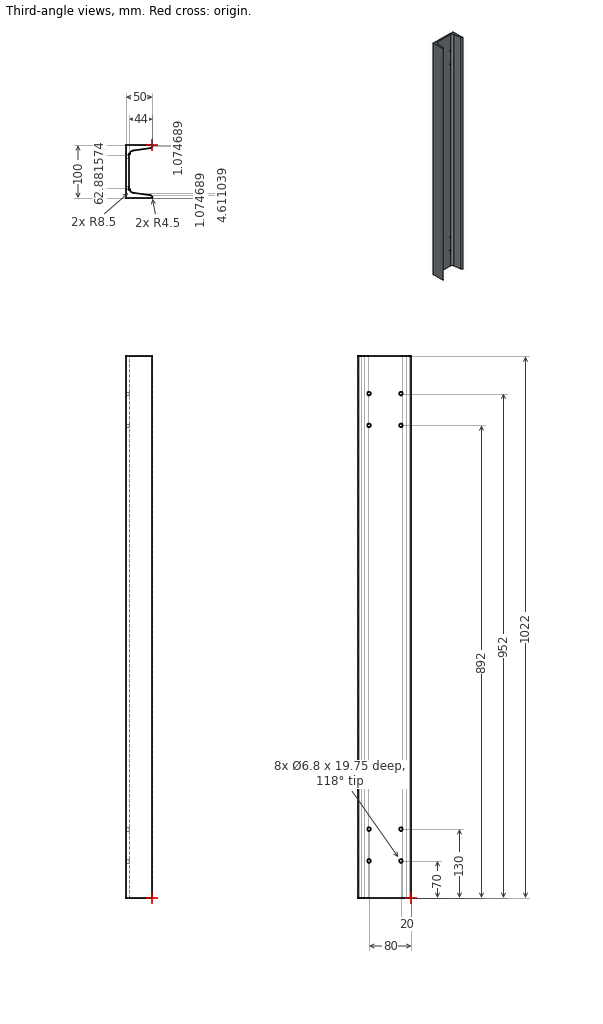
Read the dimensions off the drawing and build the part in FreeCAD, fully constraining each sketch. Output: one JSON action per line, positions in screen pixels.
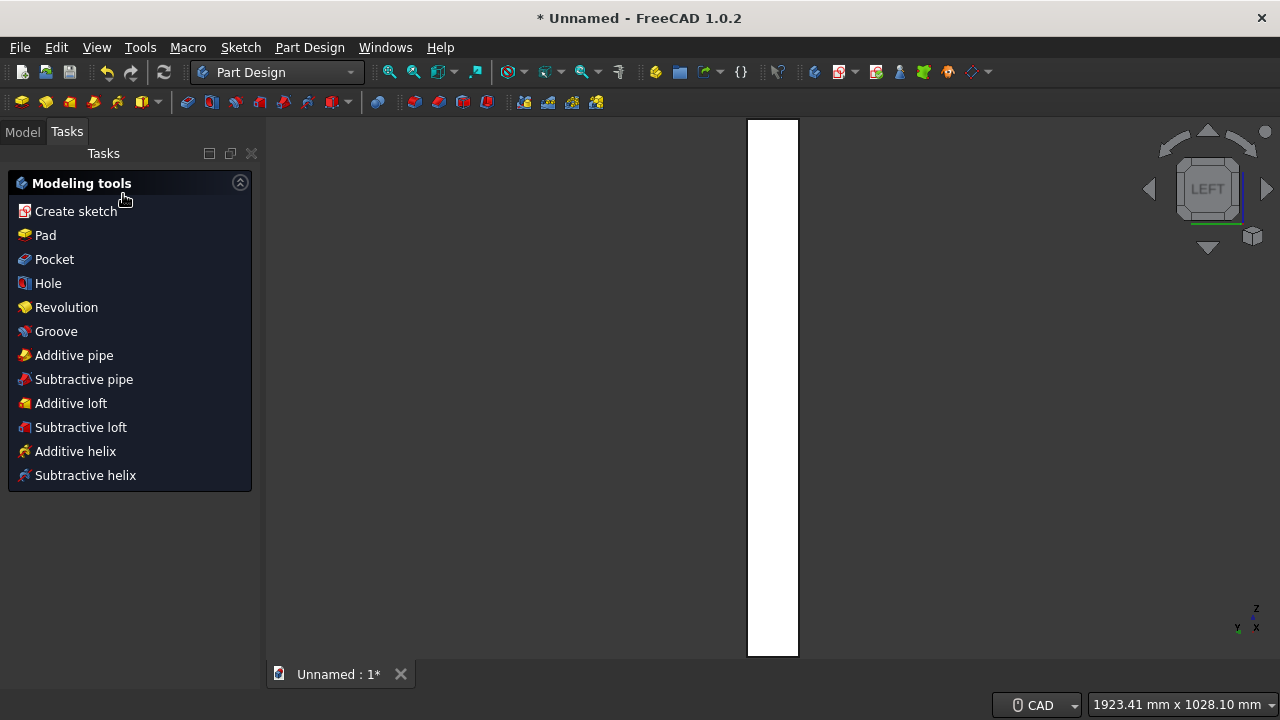
{"action": "left_click", "coordinate": [212, 102]}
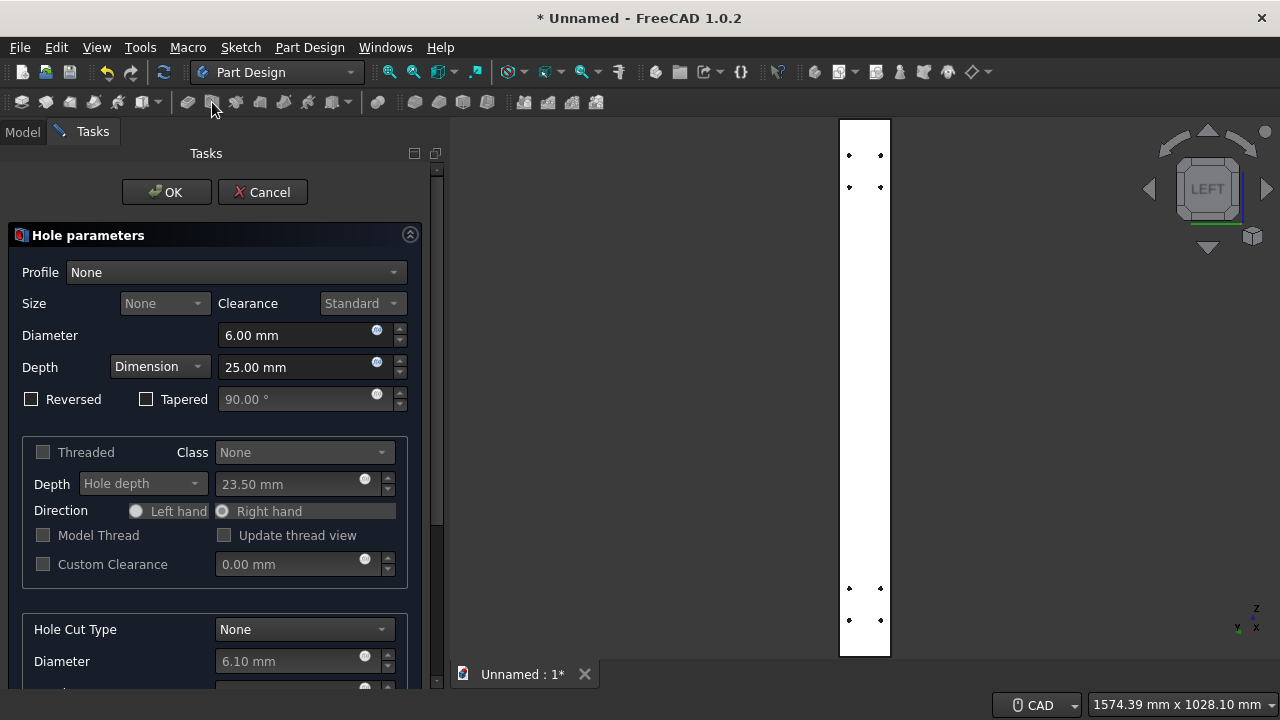
{"action": "triple_click", "coordinate": [305, 335]}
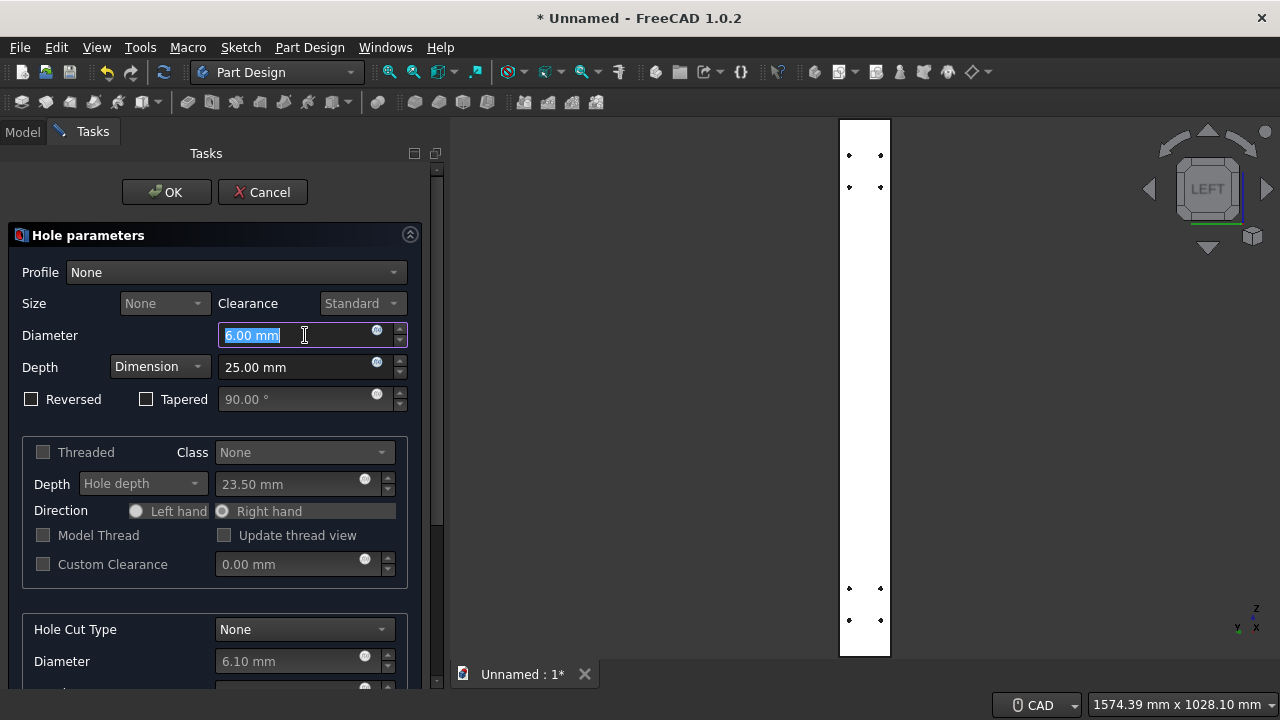
{"action": "type", "text": "6.8"}
{"action": "key", "text": "Tab"}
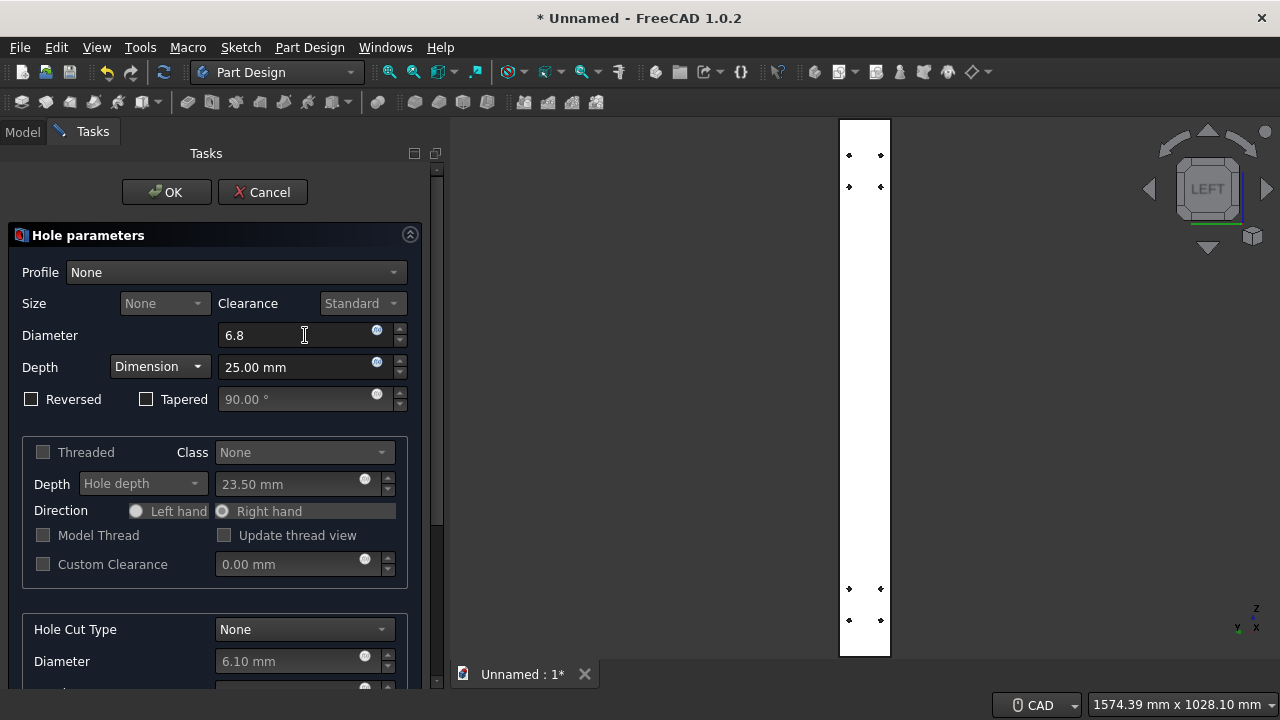
{"action": "triple_click", "coordinate": [305, 367]}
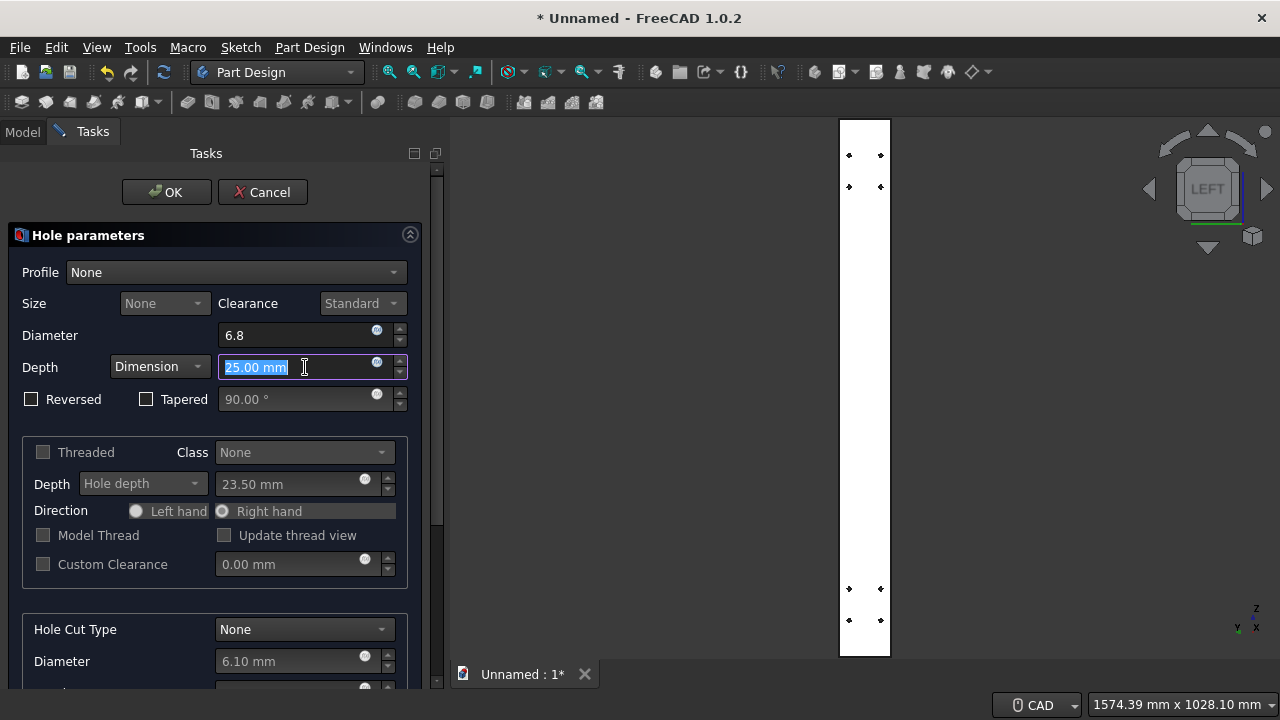
{"action": "type", "text": "19.75"}
{"action": "key", "text": "Tab"}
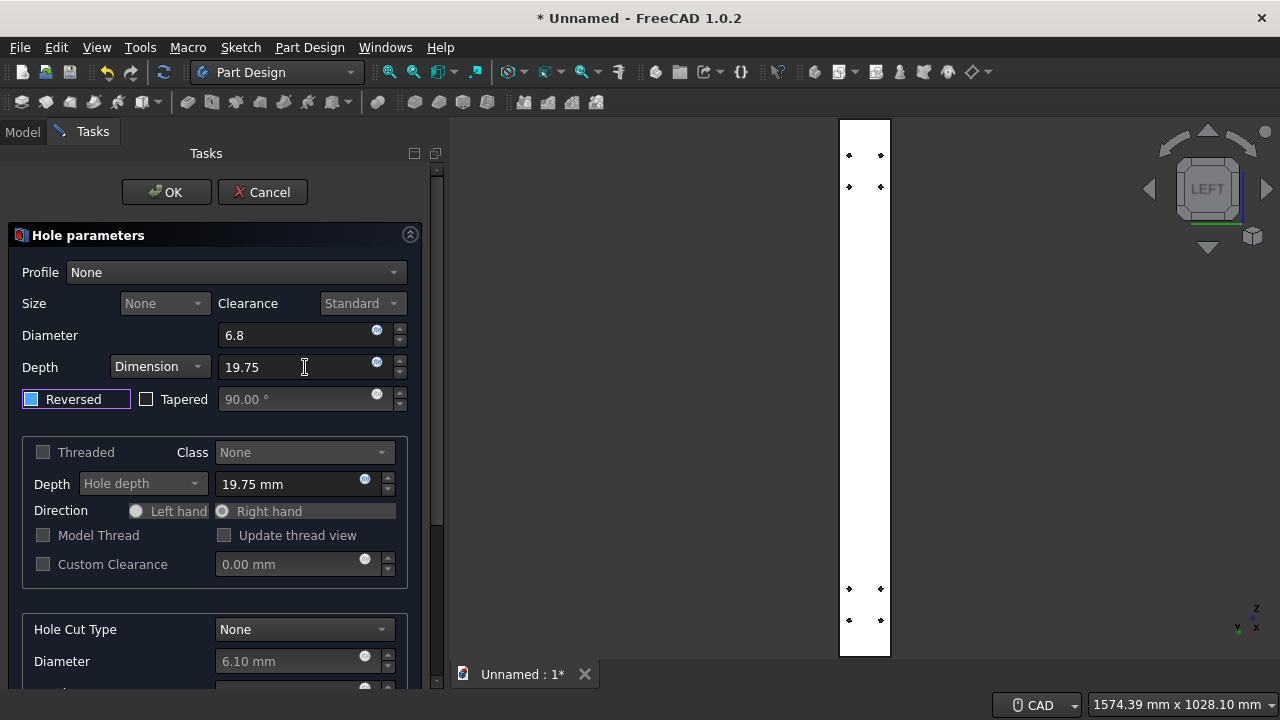
{"action": "left_click", "coordinate": [167, 192]}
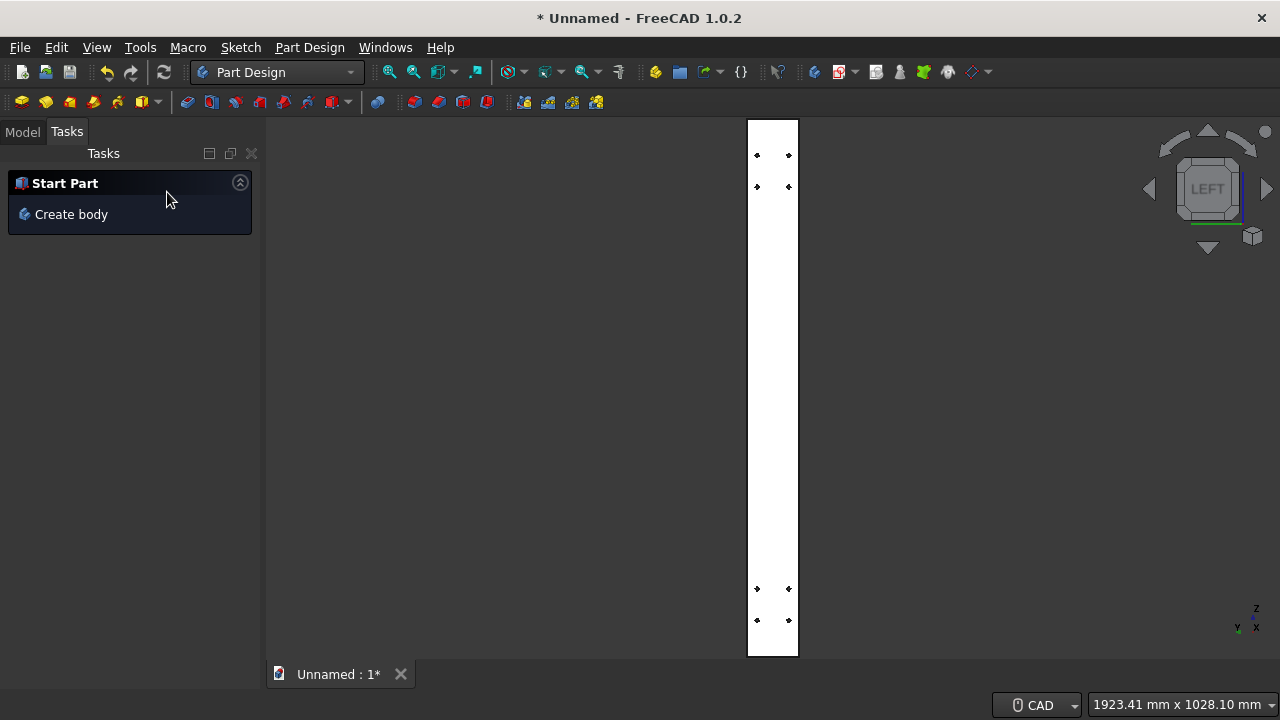
{"action": "key", "text": "0"}